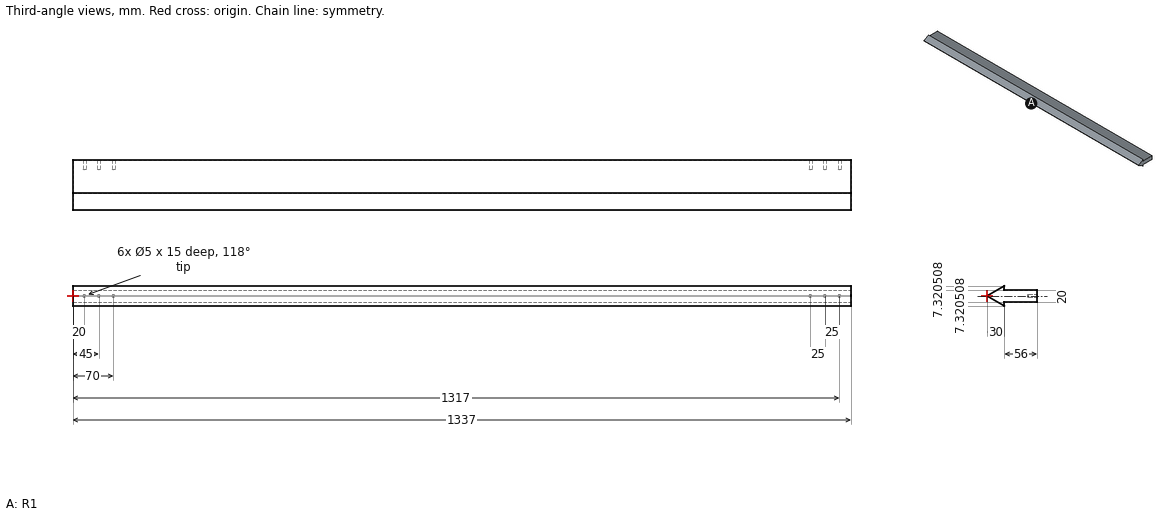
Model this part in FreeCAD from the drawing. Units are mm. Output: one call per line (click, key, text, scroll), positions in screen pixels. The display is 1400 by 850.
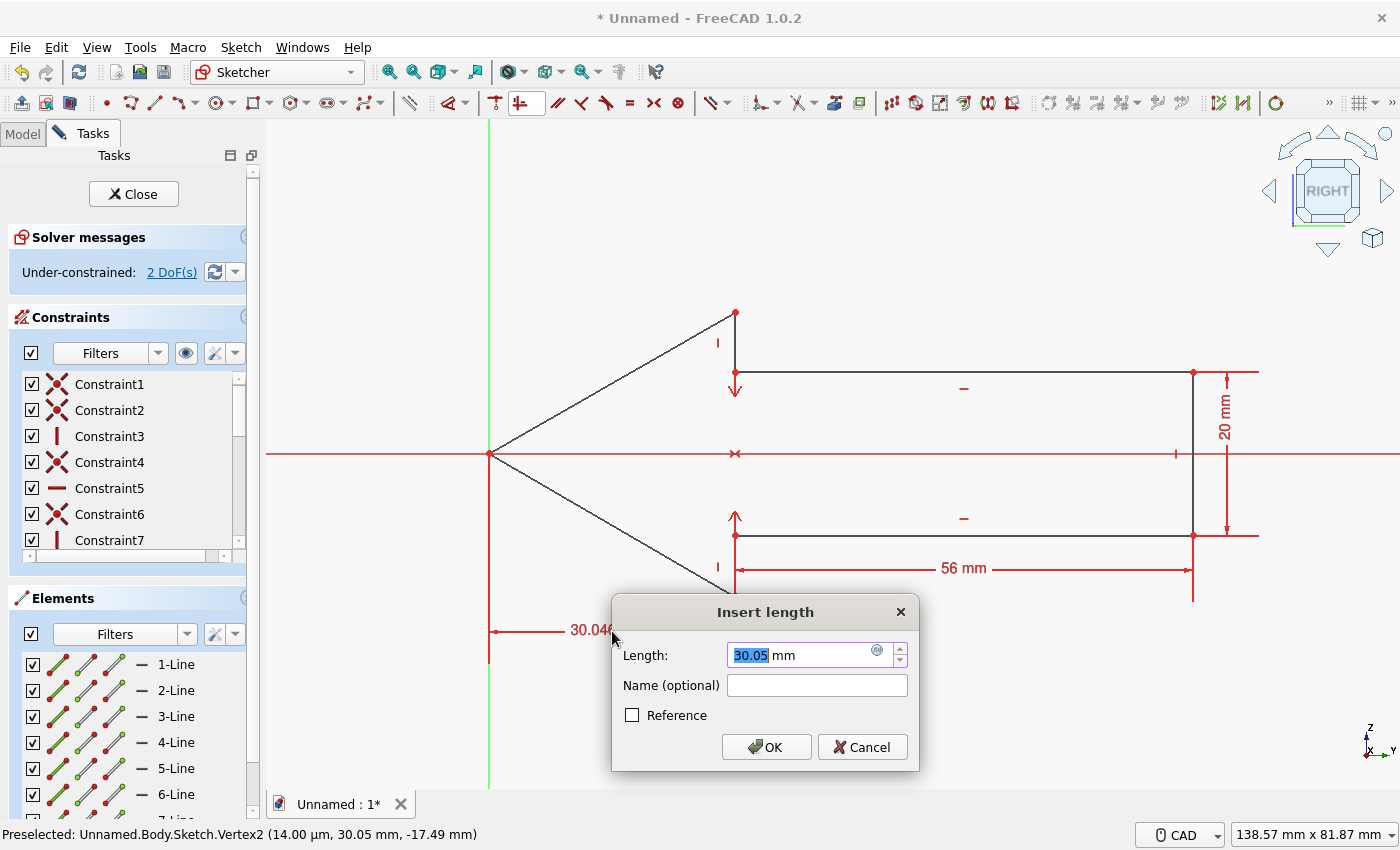
text(30)
key(Return)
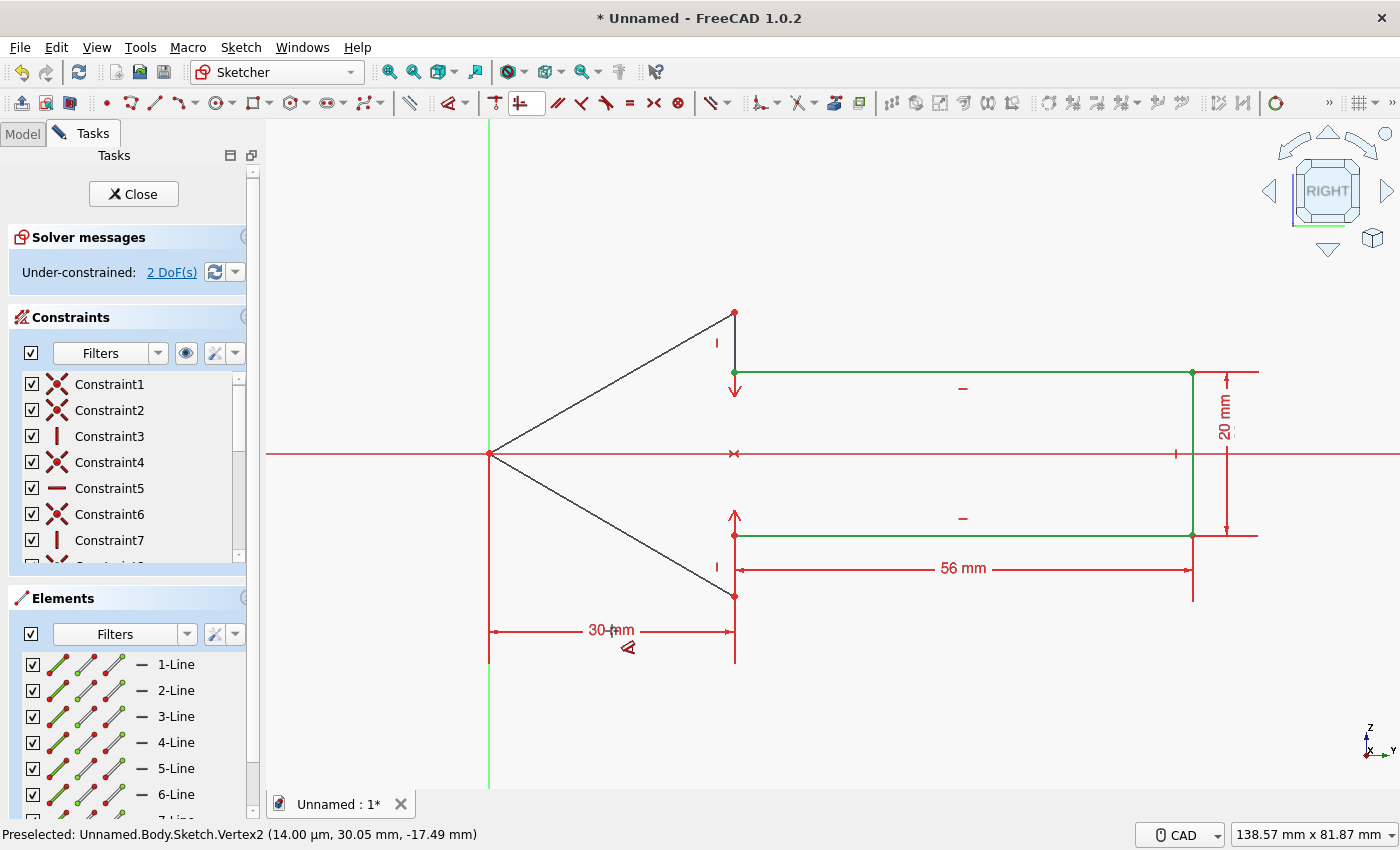
click(735, 579)
click(701, 552)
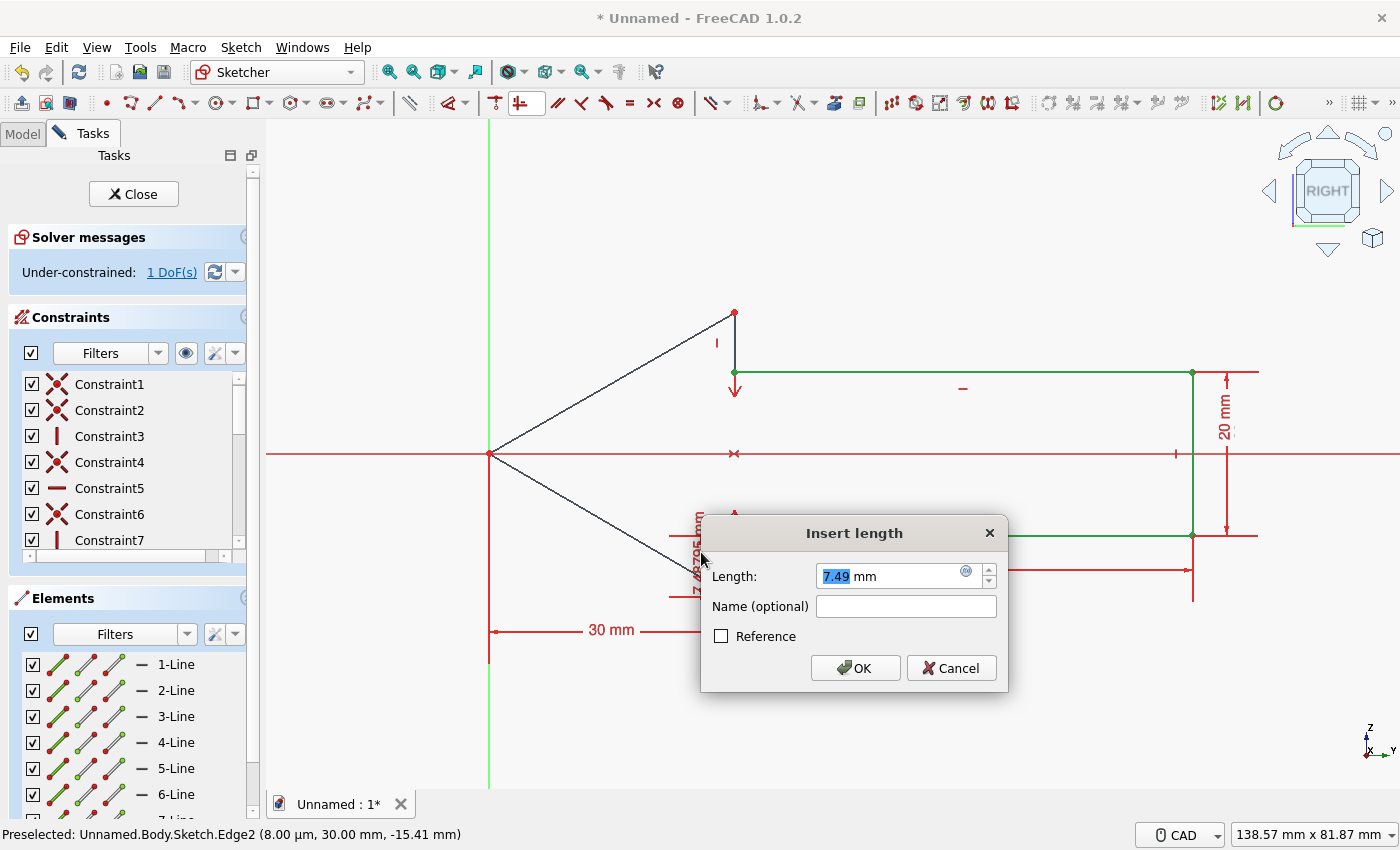
text(7.320508)
key(Return)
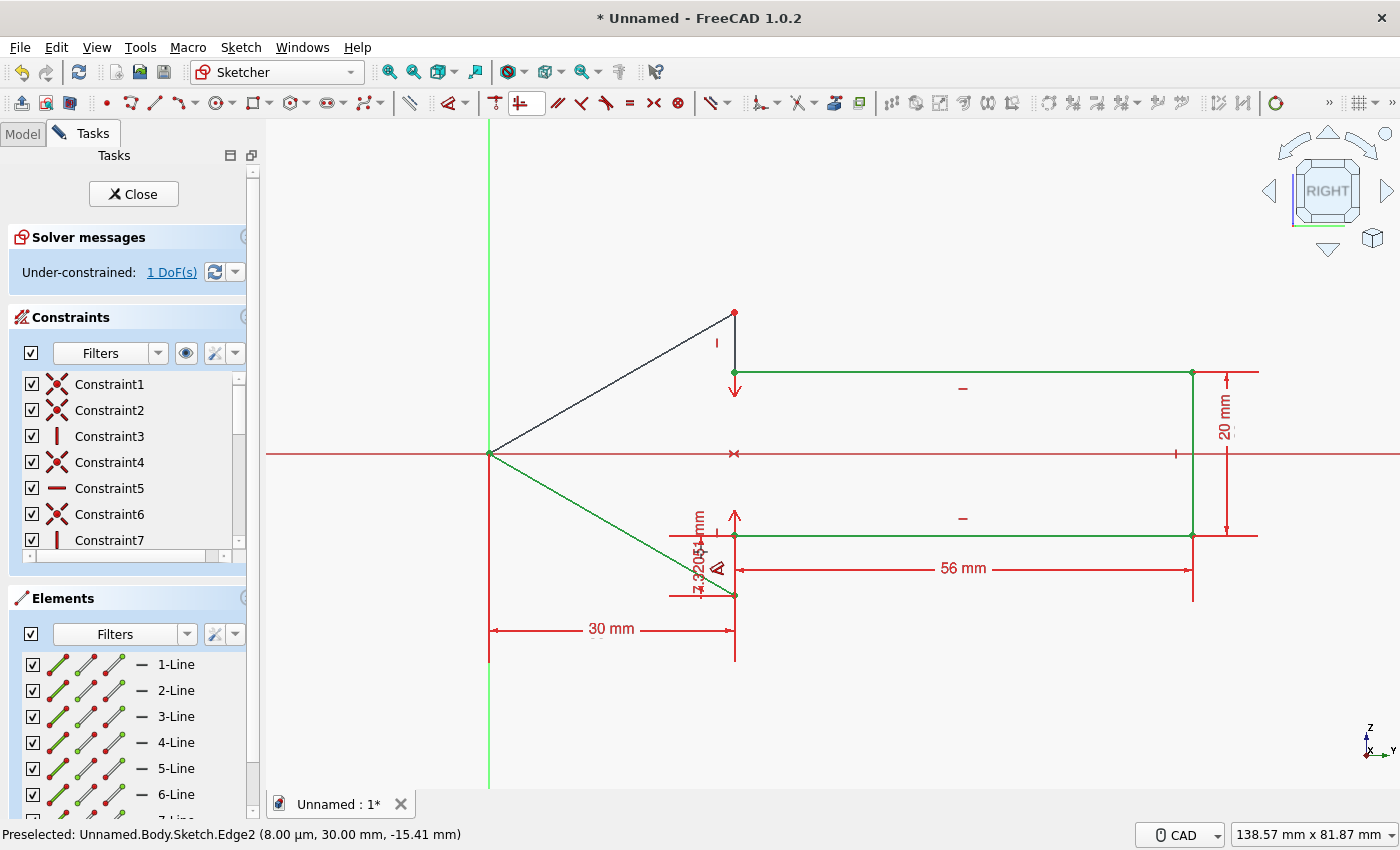
click(735, 354)
click(701, 356)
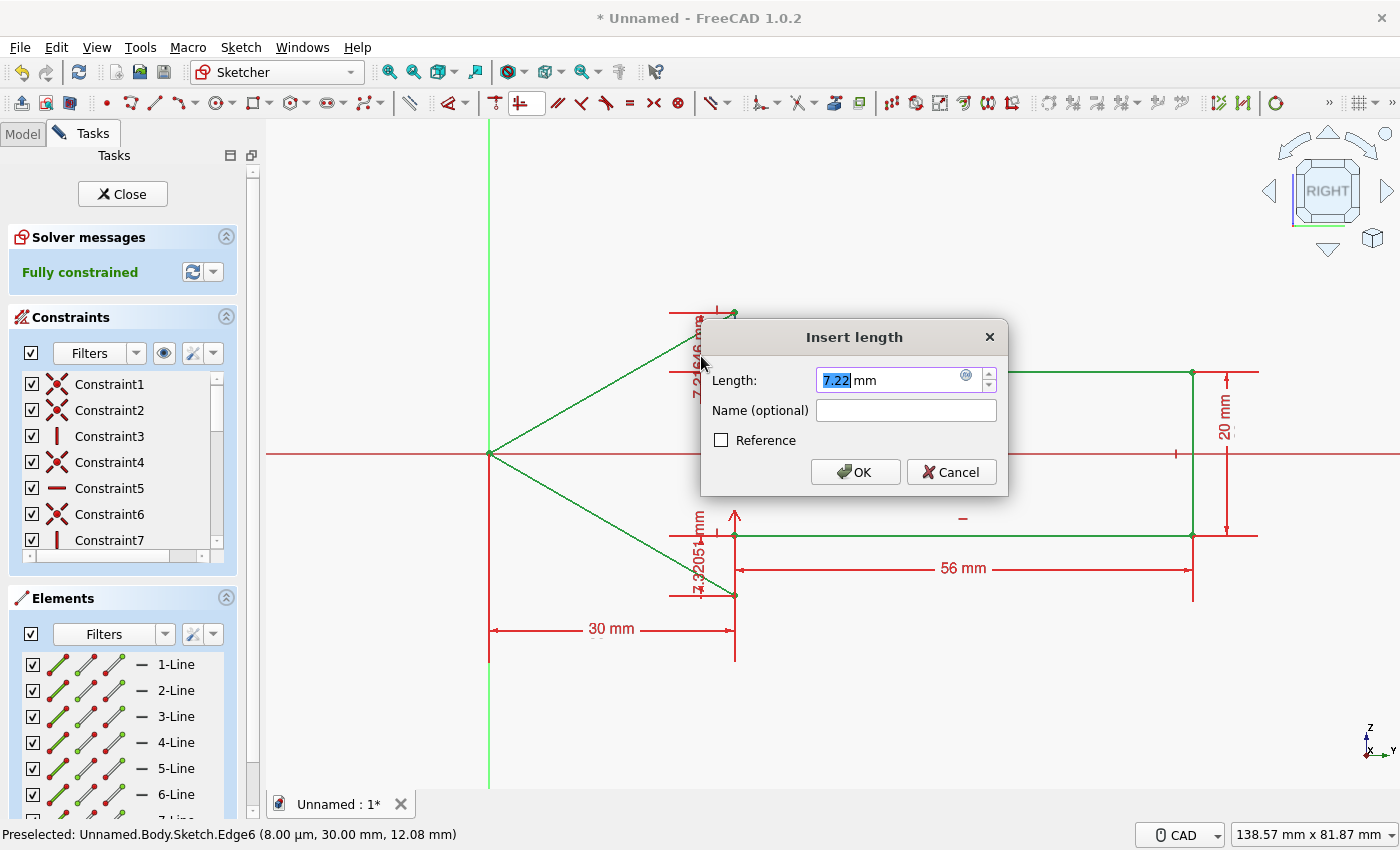
text(7.320508)
key(Return)
key(Escape)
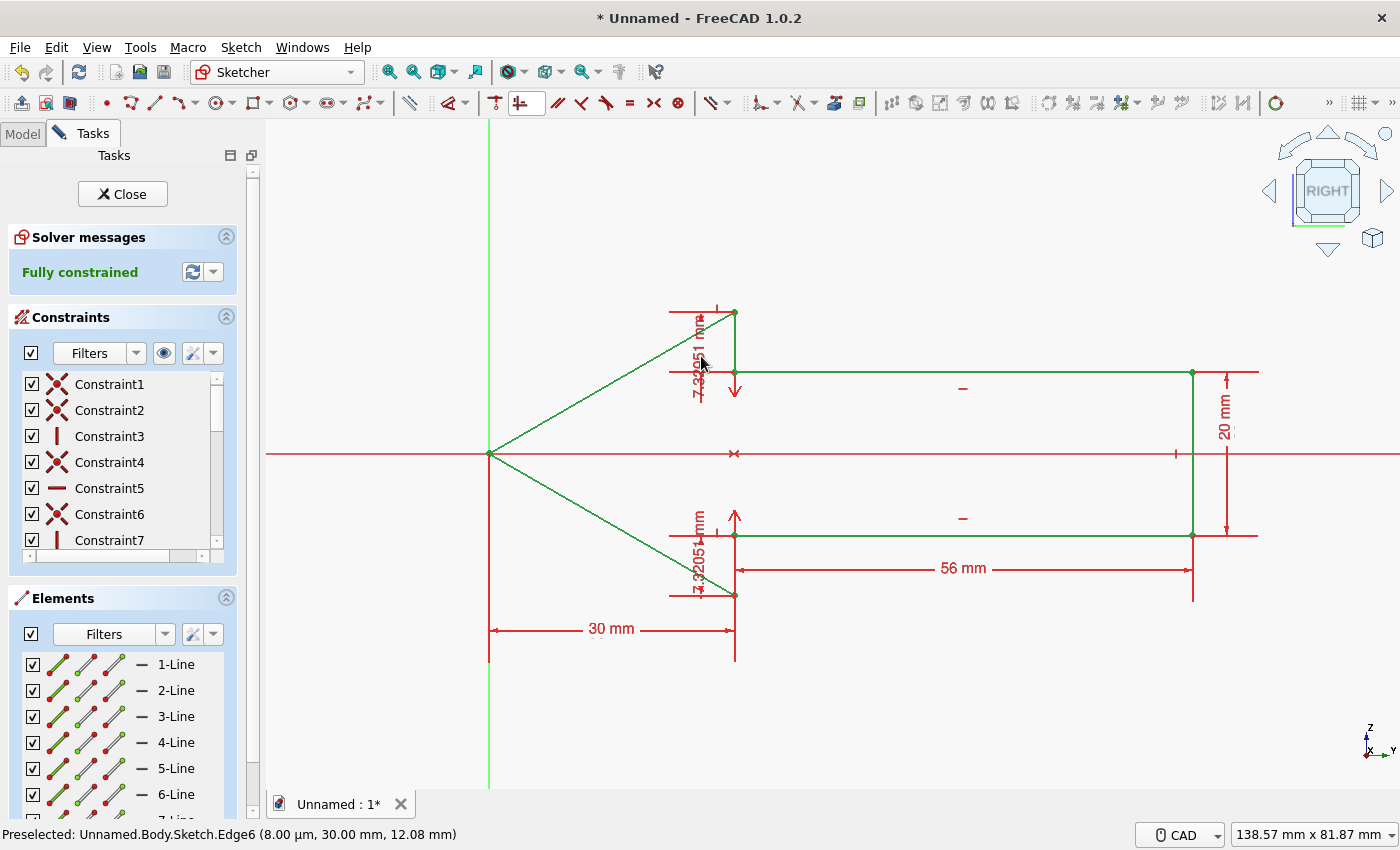
click(123, 194)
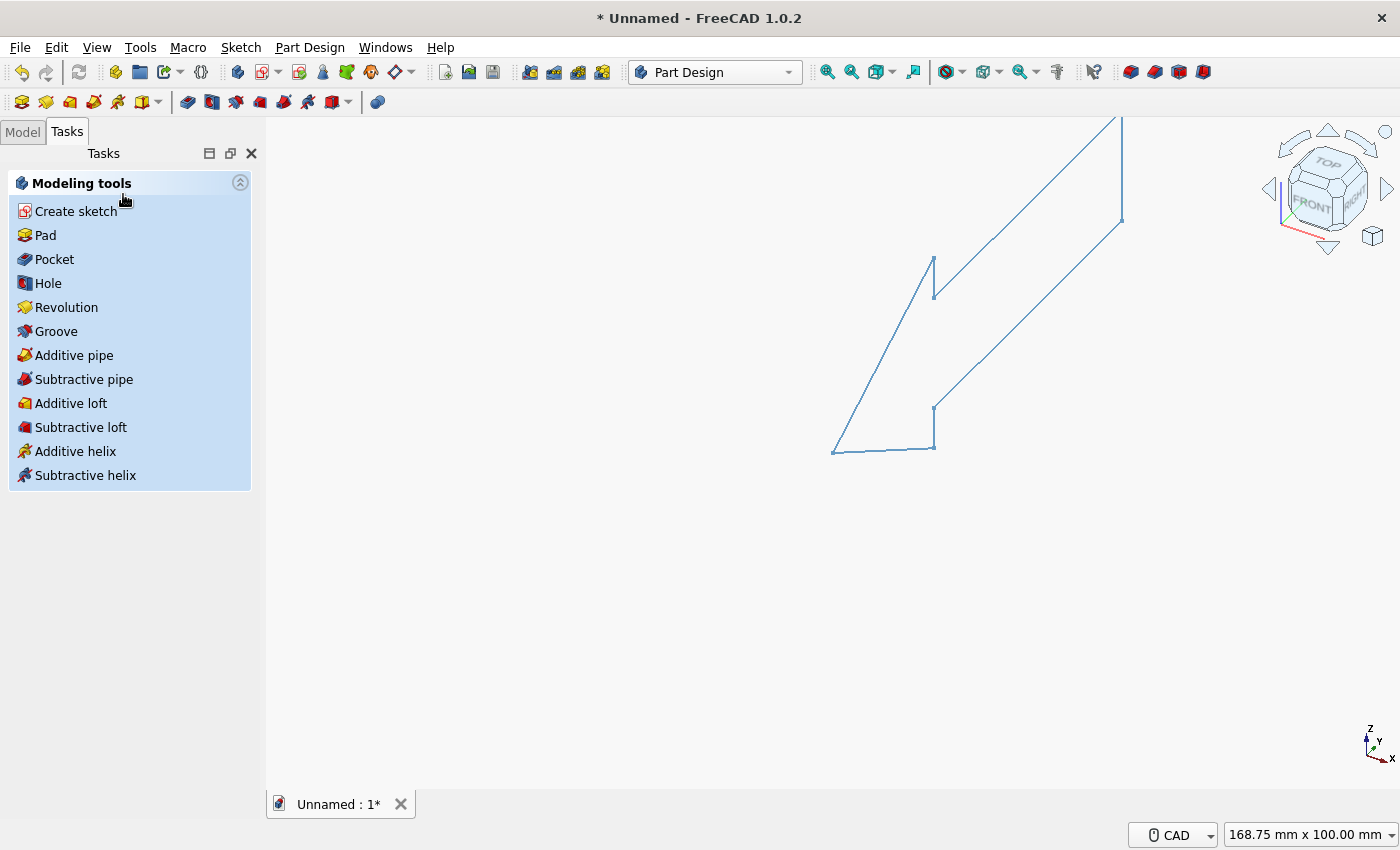
click(22, 102)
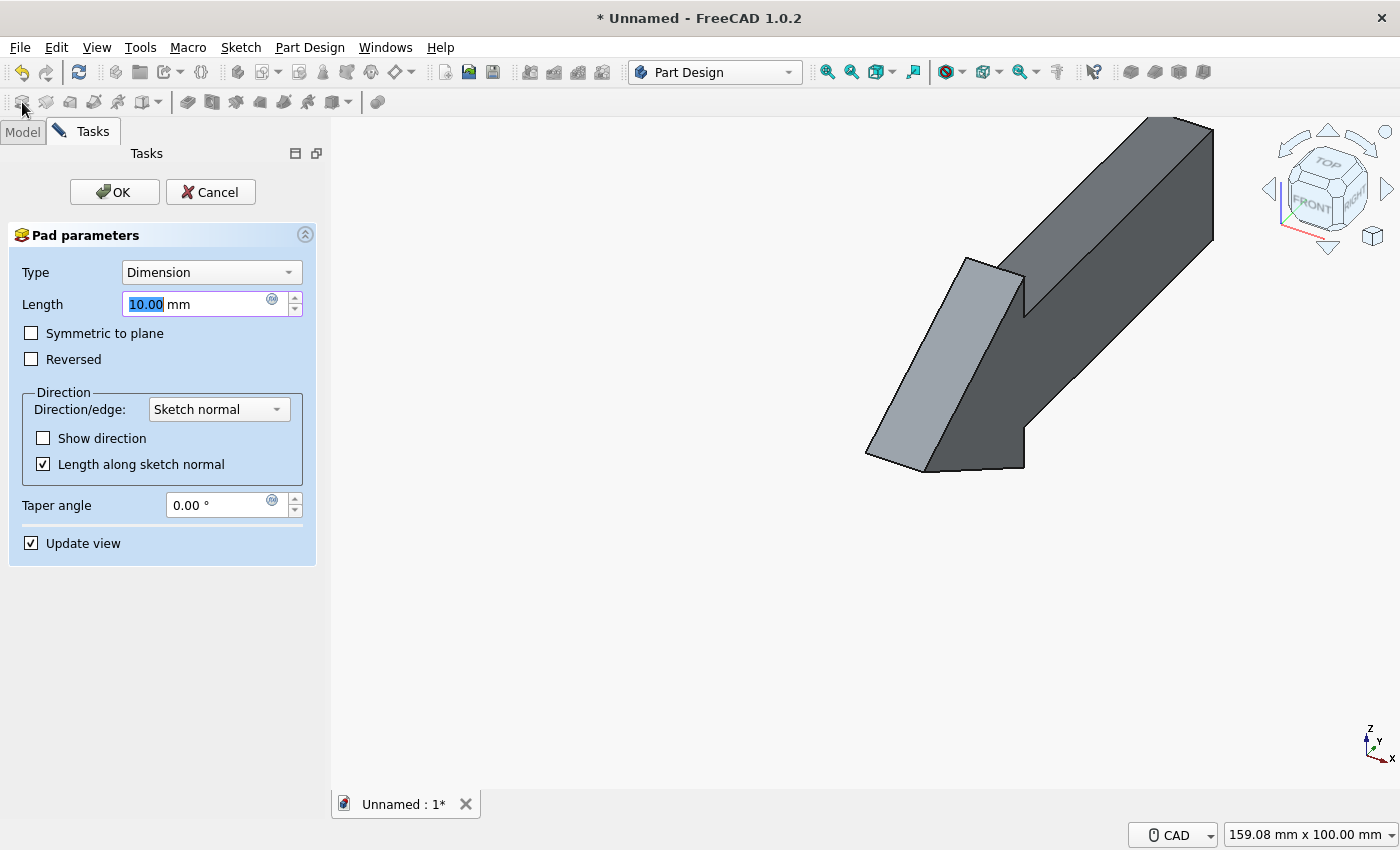
text(1337)
key(Tab)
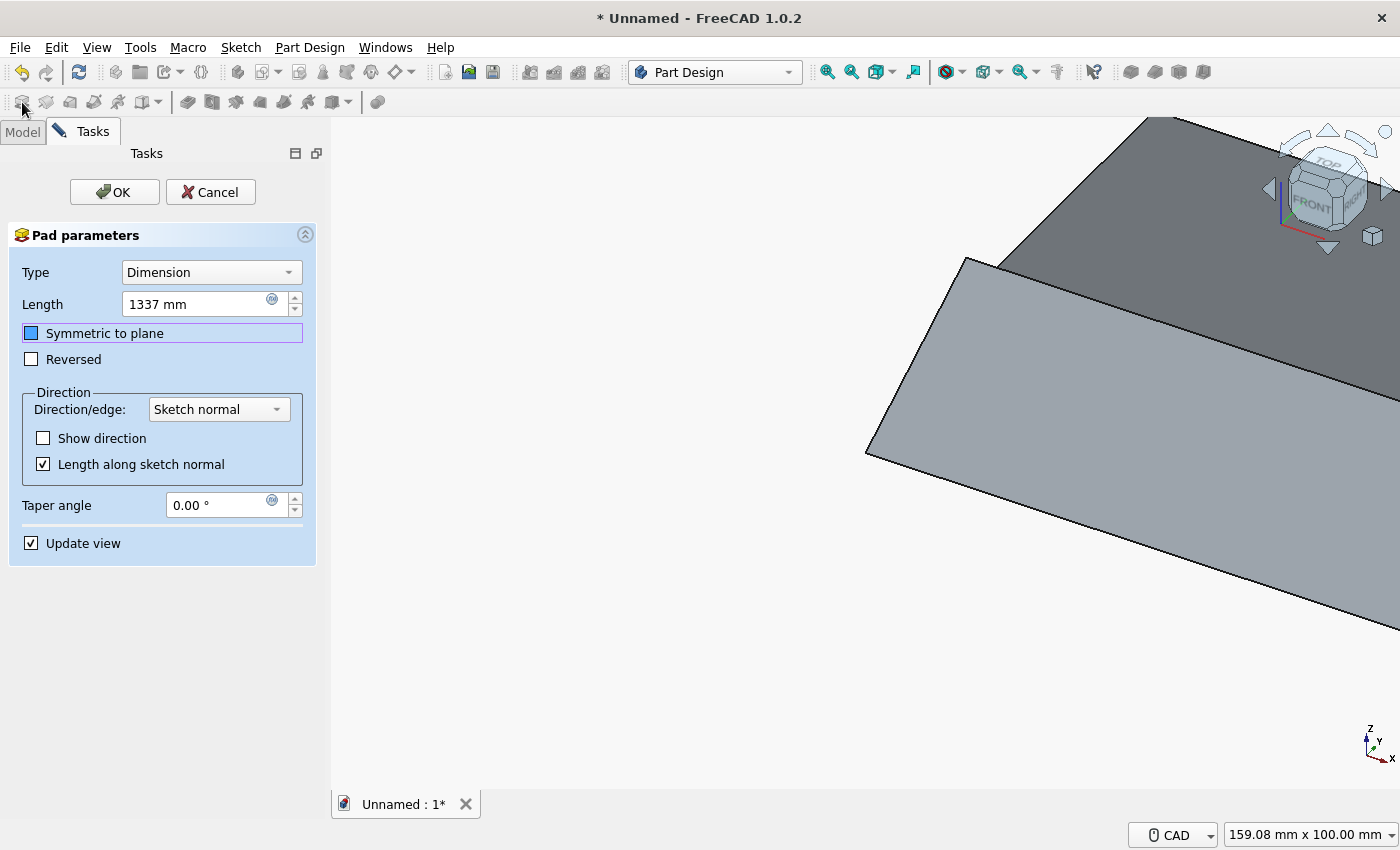
click(115, 192)